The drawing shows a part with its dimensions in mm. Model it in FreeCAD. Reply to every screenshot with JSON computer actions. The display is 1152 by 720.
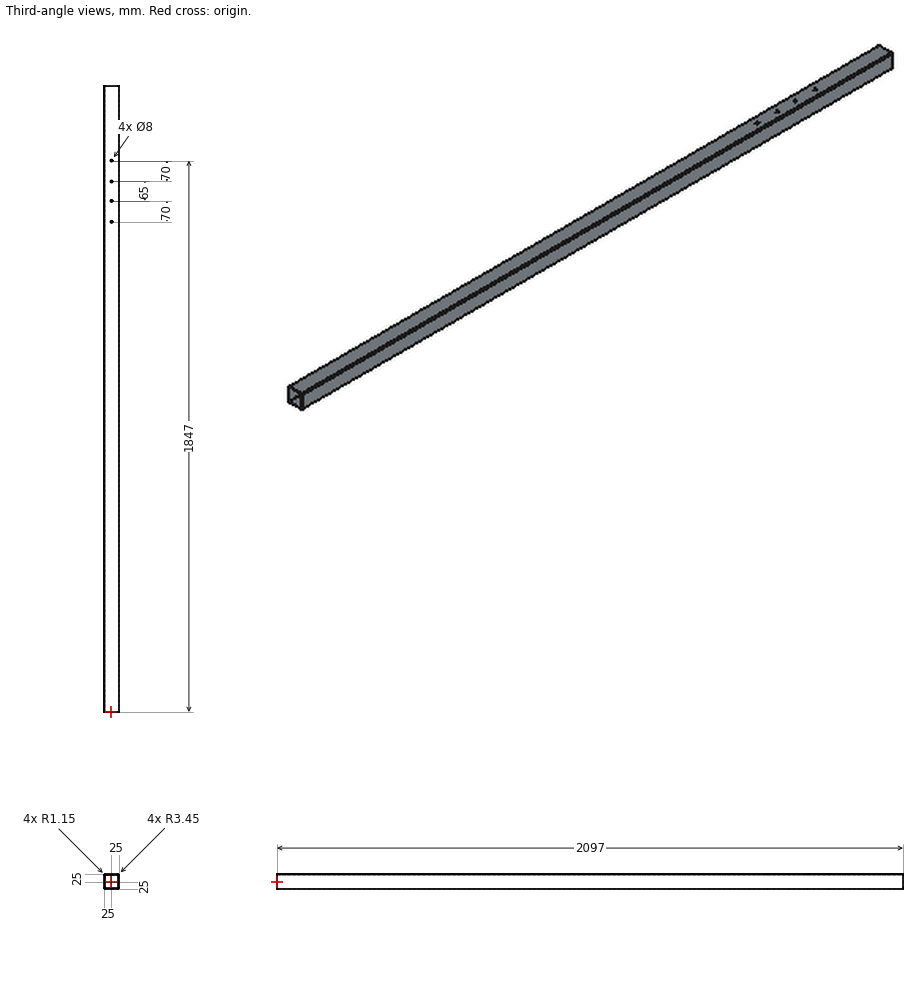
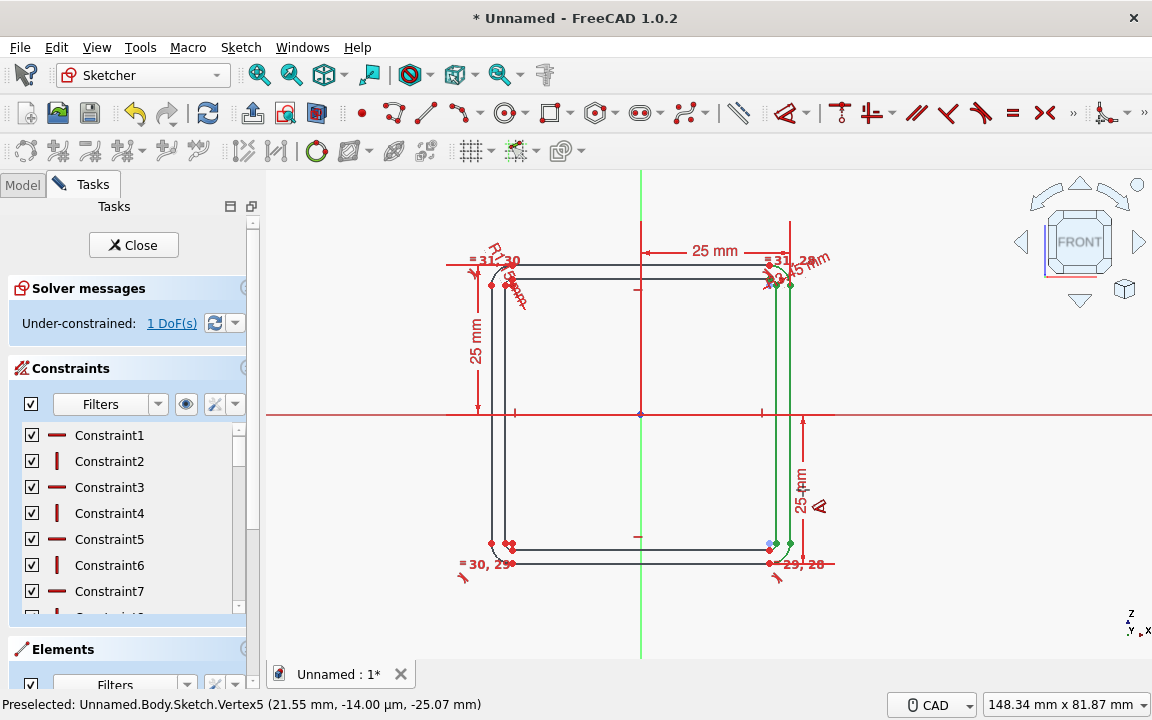
{"action": "left_click", "coordinate": [492, 543]}
{"action": "left_click", "coordinate": [566, 577]}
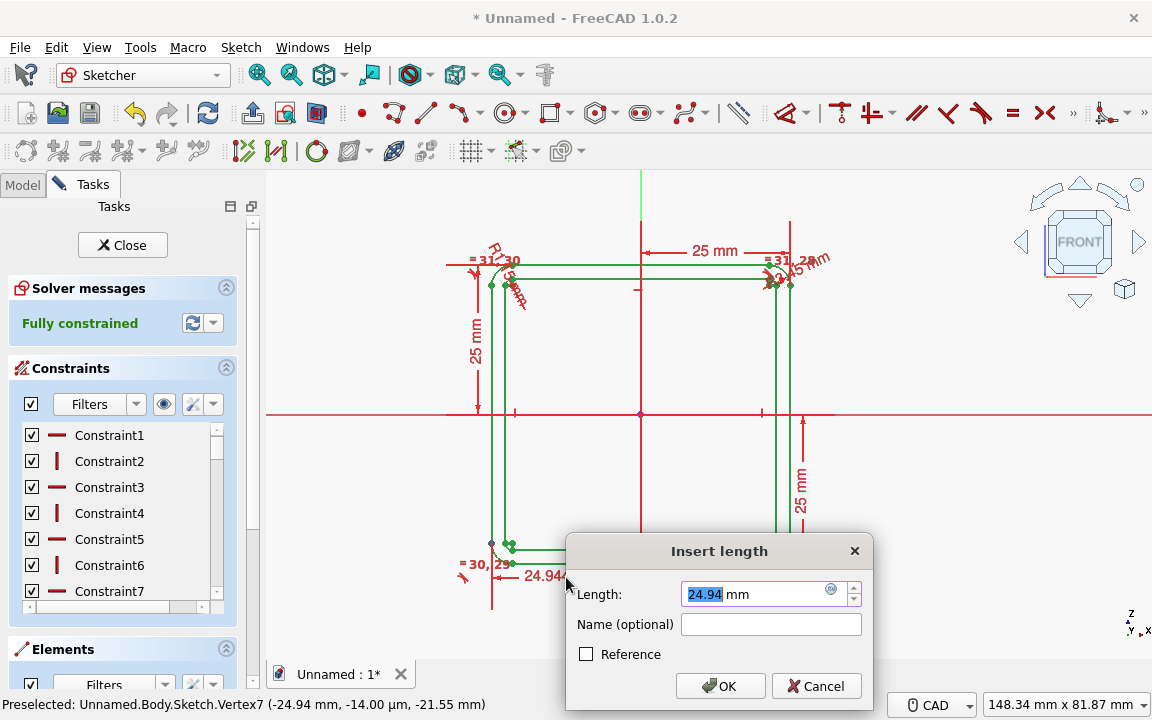
{"action": "type", "text": "25"}
{"action": "key", "text": "Return"}
{"action": "key", "text": "Escape"}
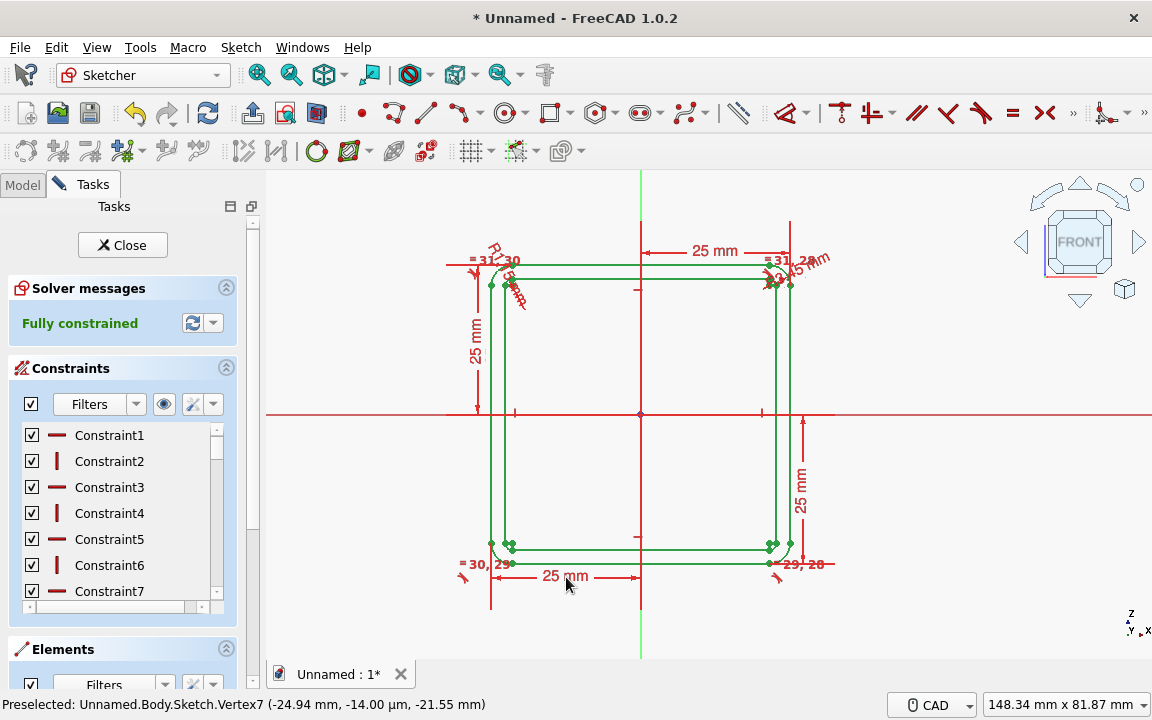
{"action": "left_click", "coordinate": [123, 245]}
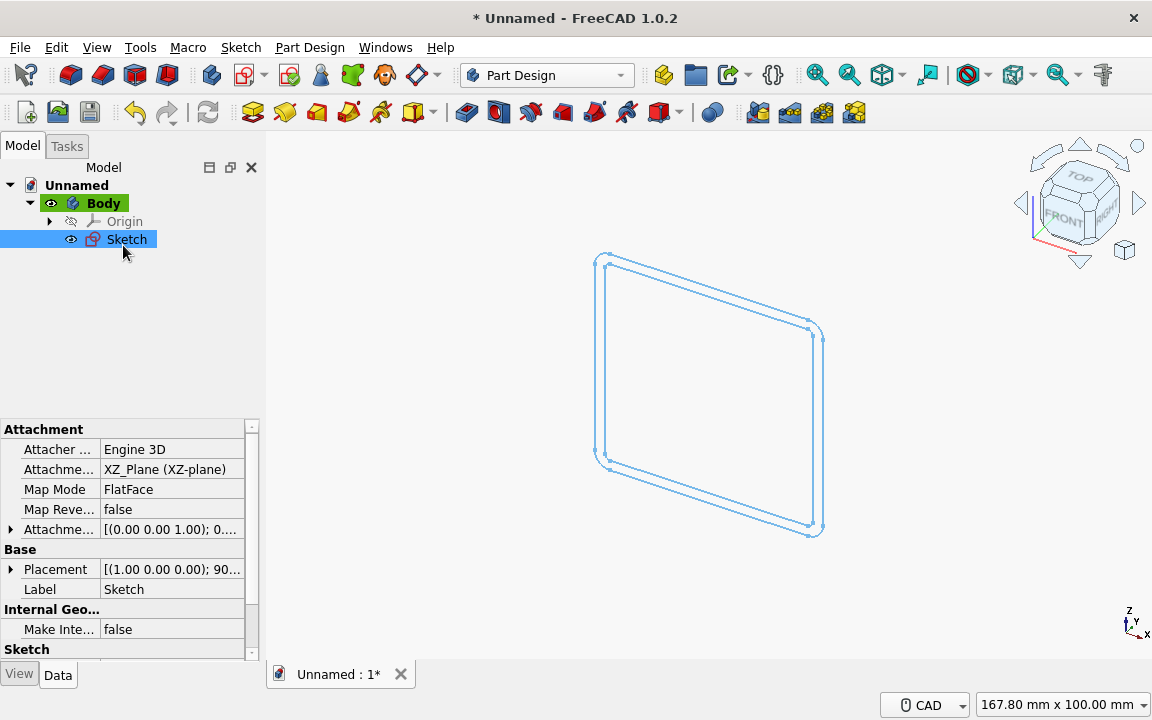
{"action": "left_click", "coordinate": [254, 112]}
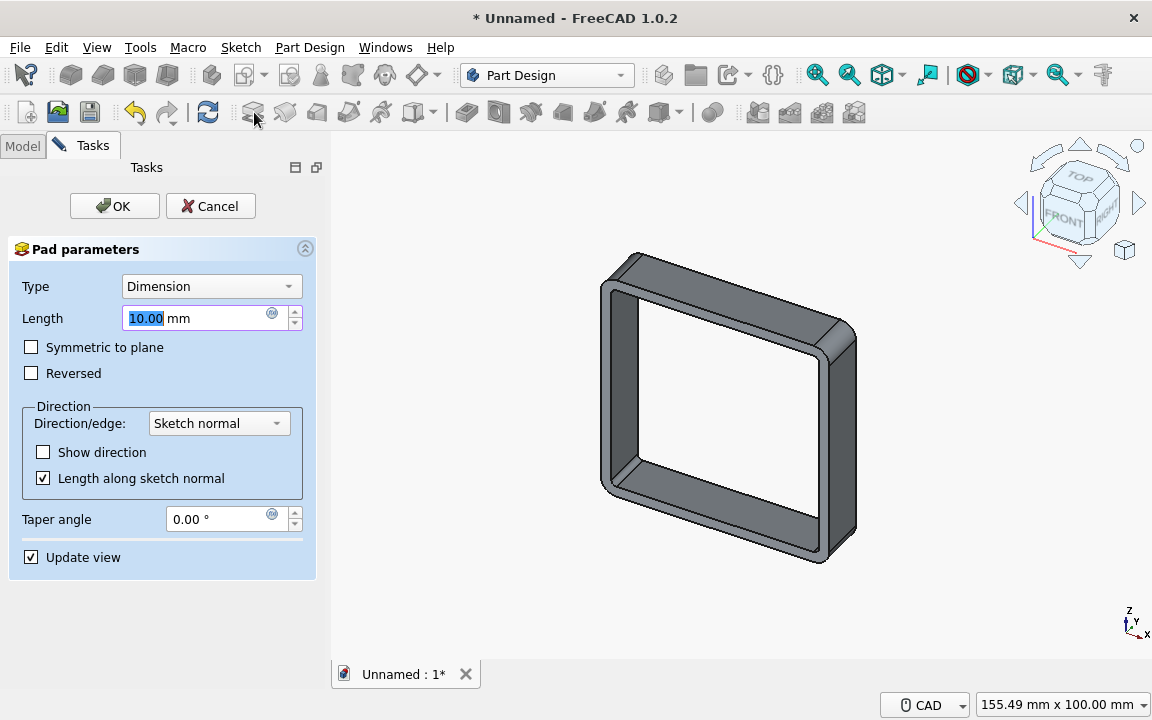
{"action": "type", "text": "2097"}
{"action": "key", "text": "Tab"}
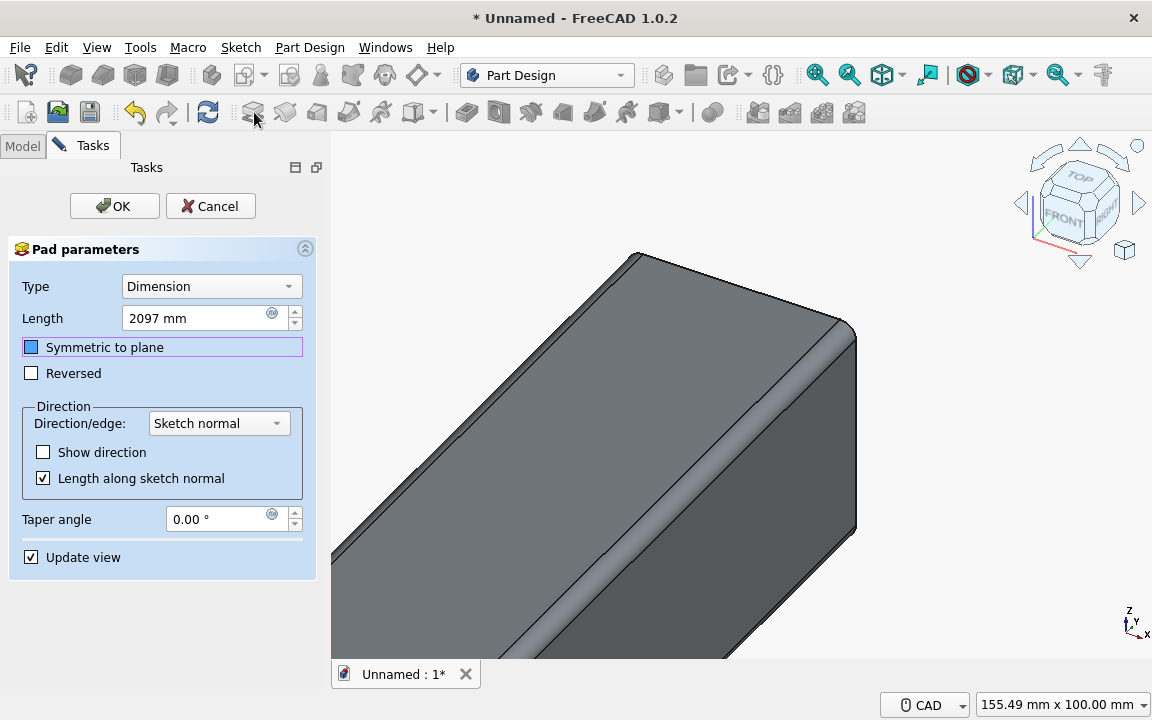
{"action": "left_click", "coordinate": [30, 373]}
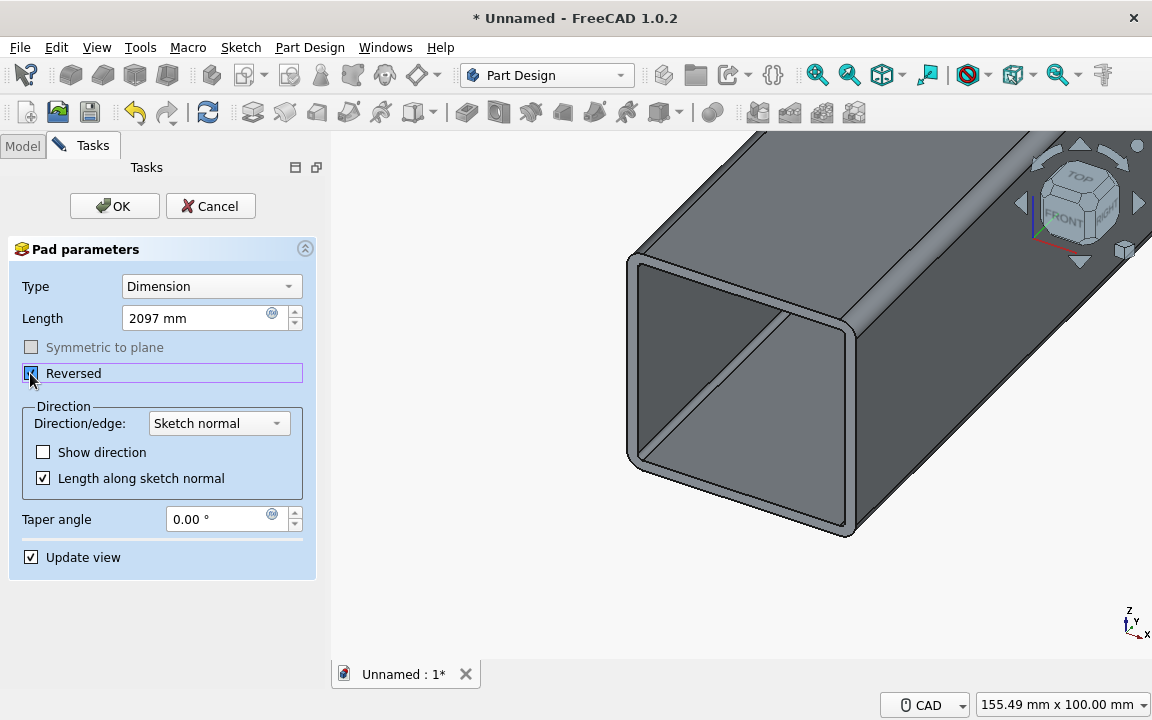
{"action": "left_click", "coordinate": [115, 206]}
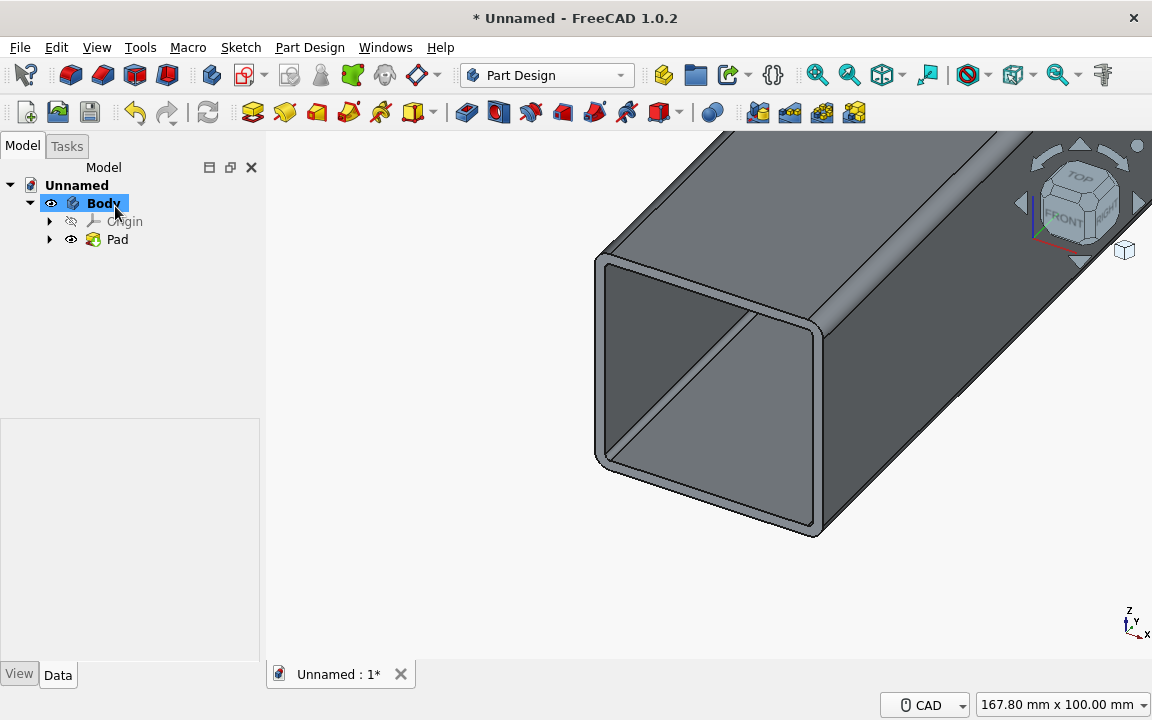
{"action": "left_click", "coordinate": [818, 76]}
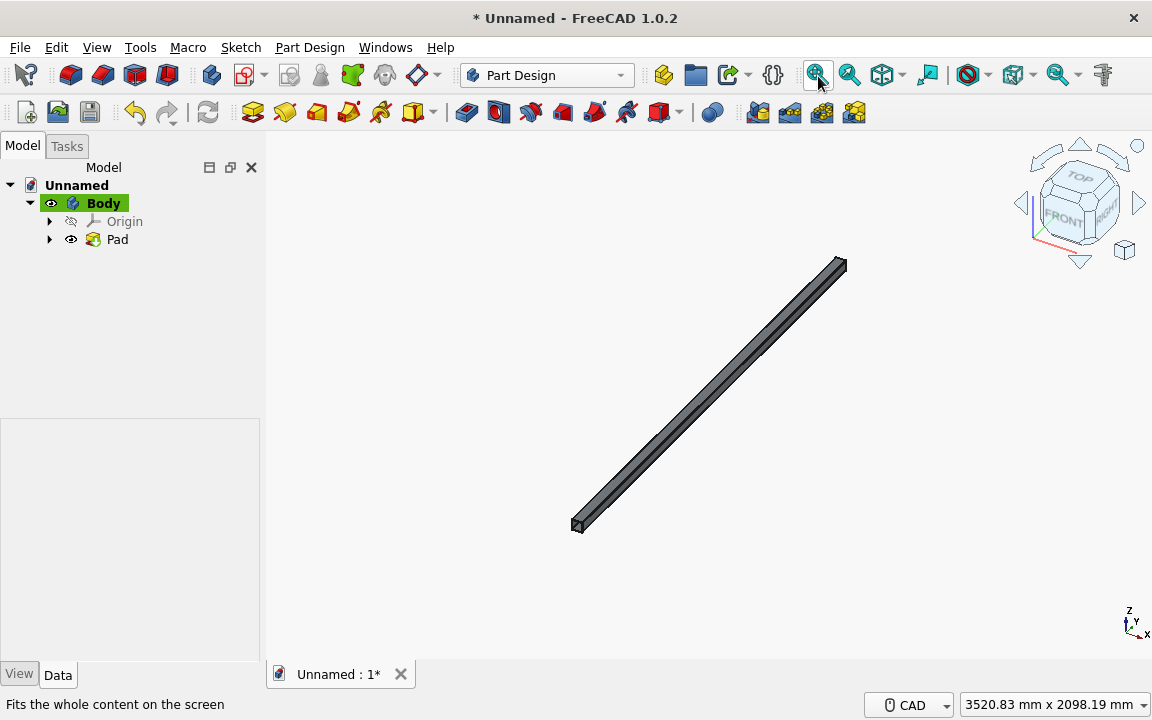
{"action": "key", "text": "5"}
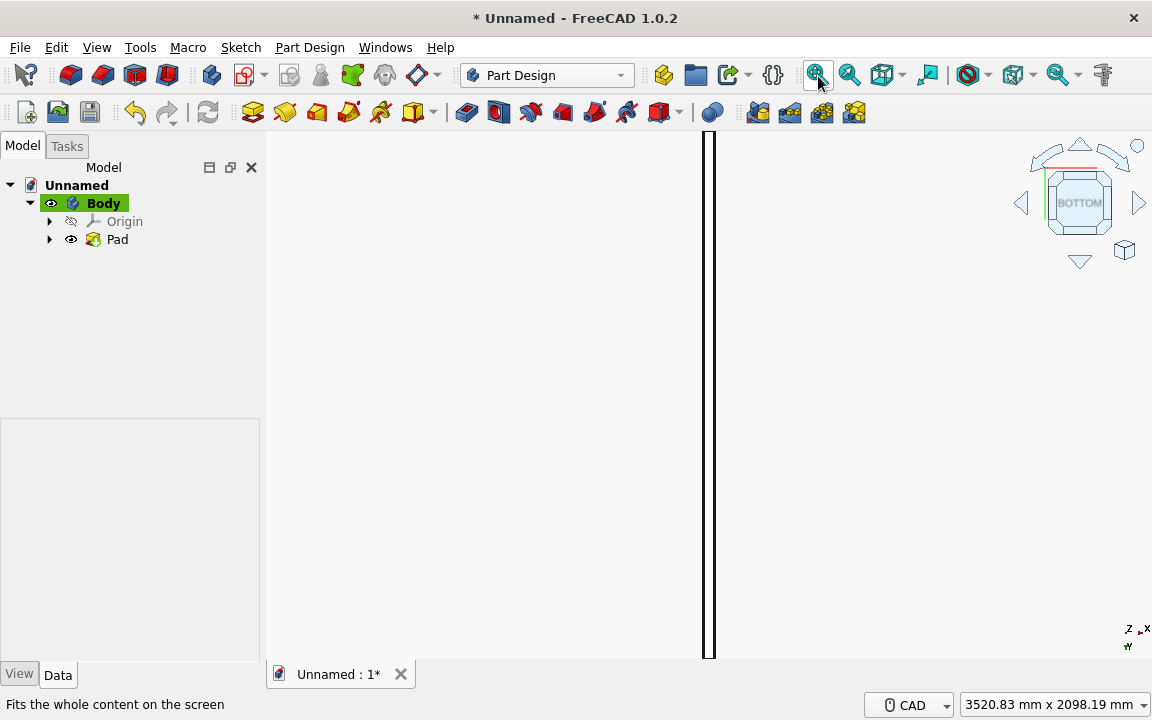
{"action": "left_click", "coordinate": [818, 76]}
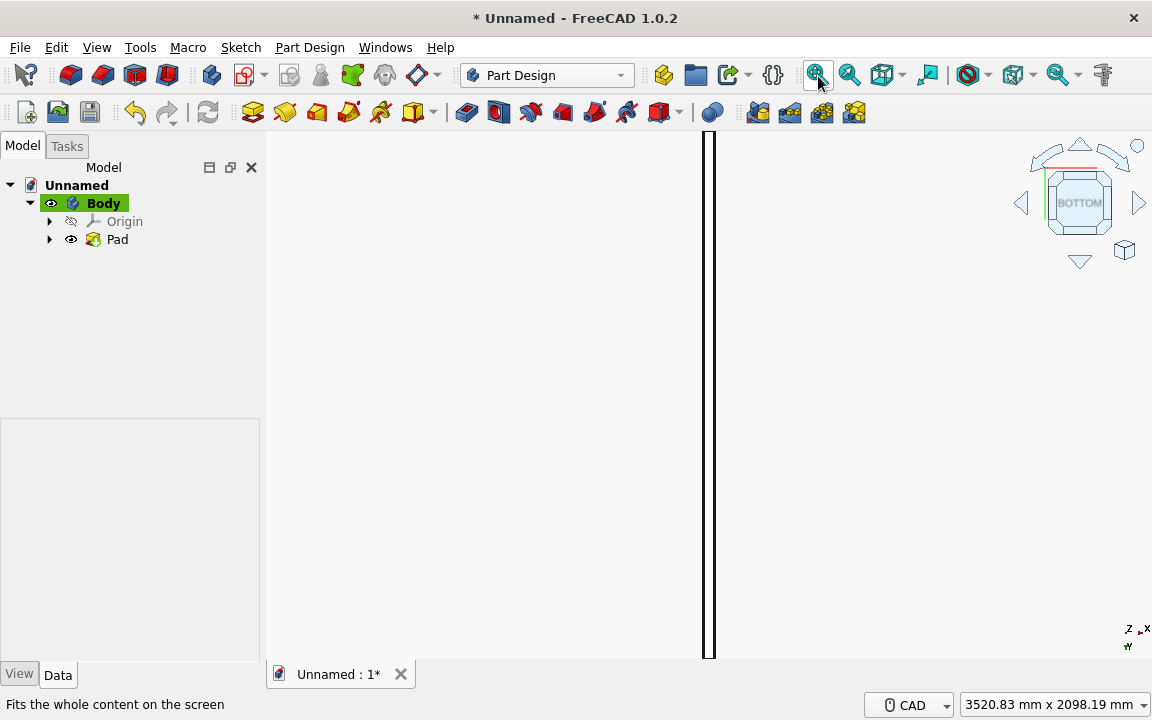
{"action": "scroll", "coordinate": [709, 620], "scroll_direction": "up", "scroll_amount": 4}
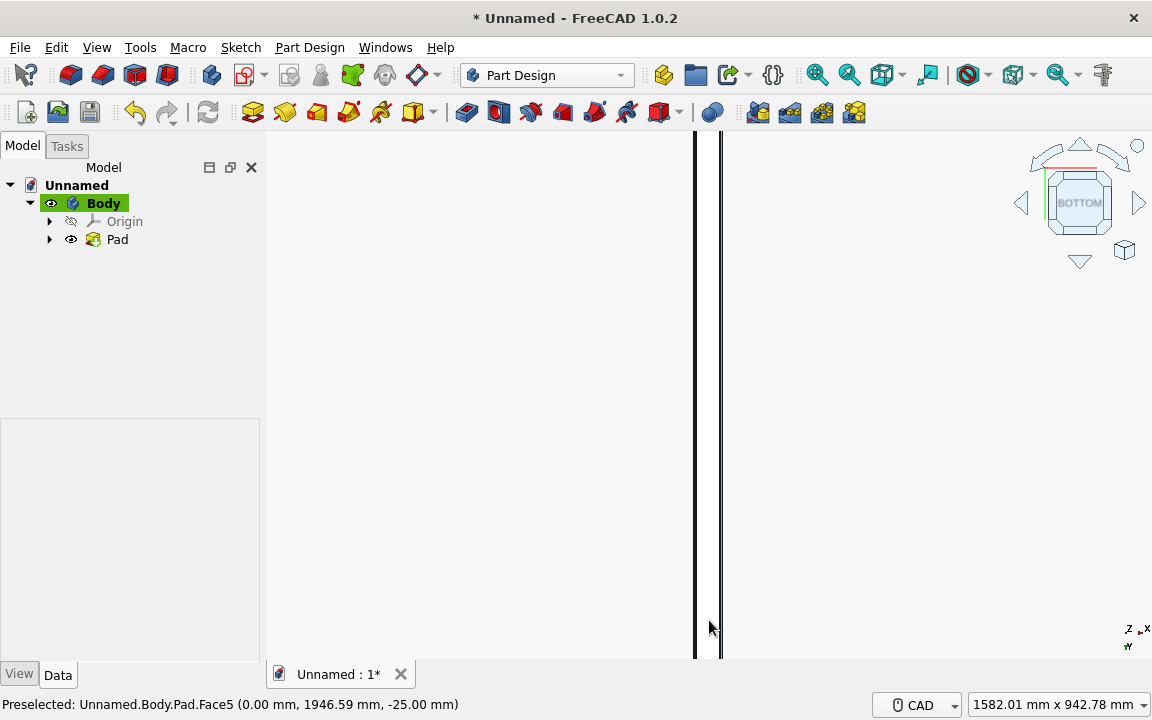
{"action": "left_click", "coordinate": [708, 620]}